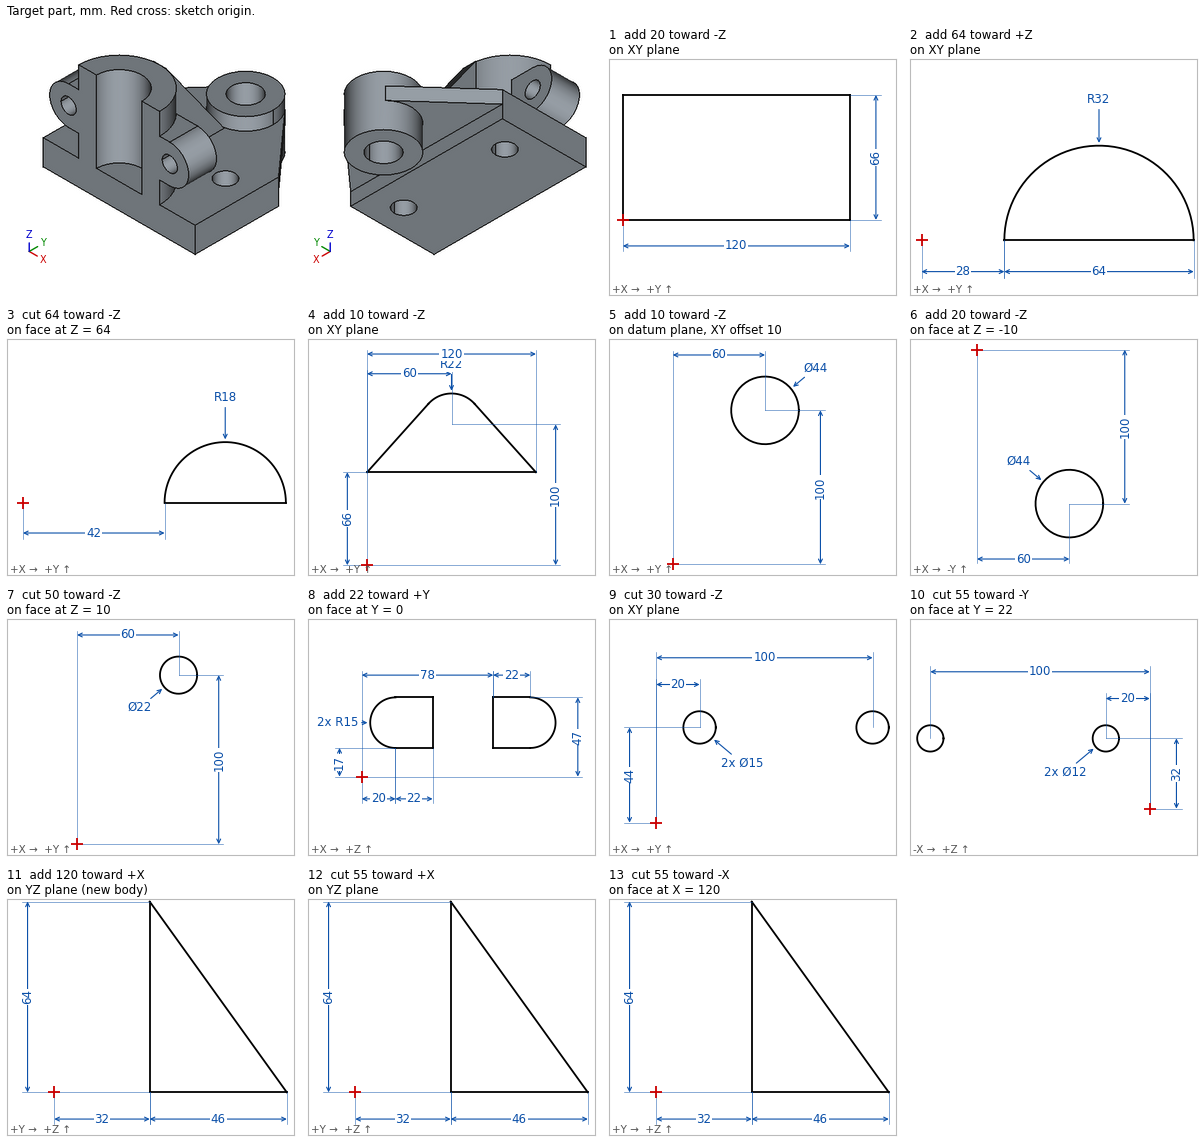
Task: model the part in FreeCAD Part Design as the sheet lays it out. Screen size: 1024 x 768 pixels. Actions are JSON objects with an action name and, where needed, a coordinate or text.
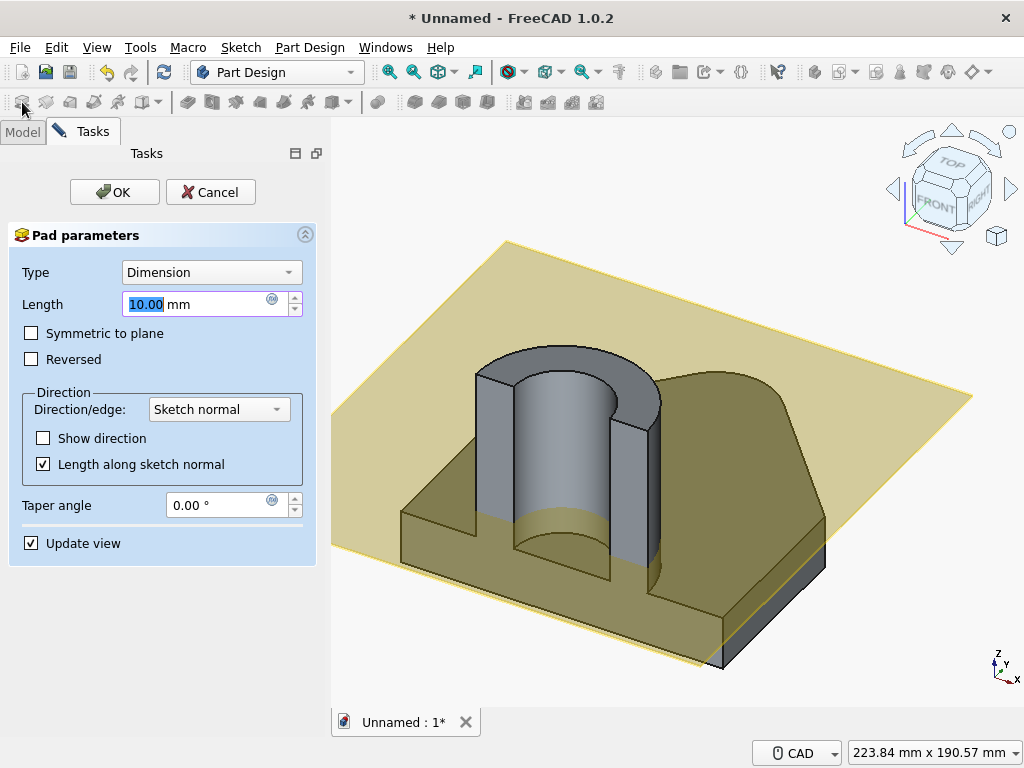
{"action": "type", "text": "10"}
{"action": "key", "text": "Tab"}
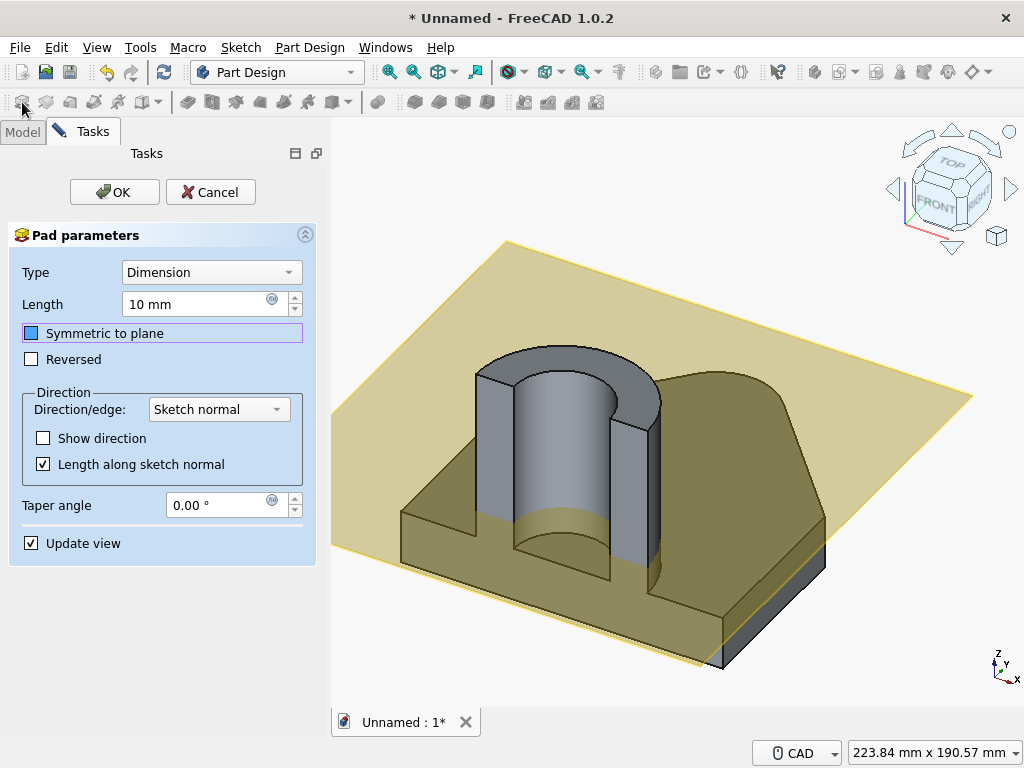
{"action": "left_click", "coordinate": [30, 359]}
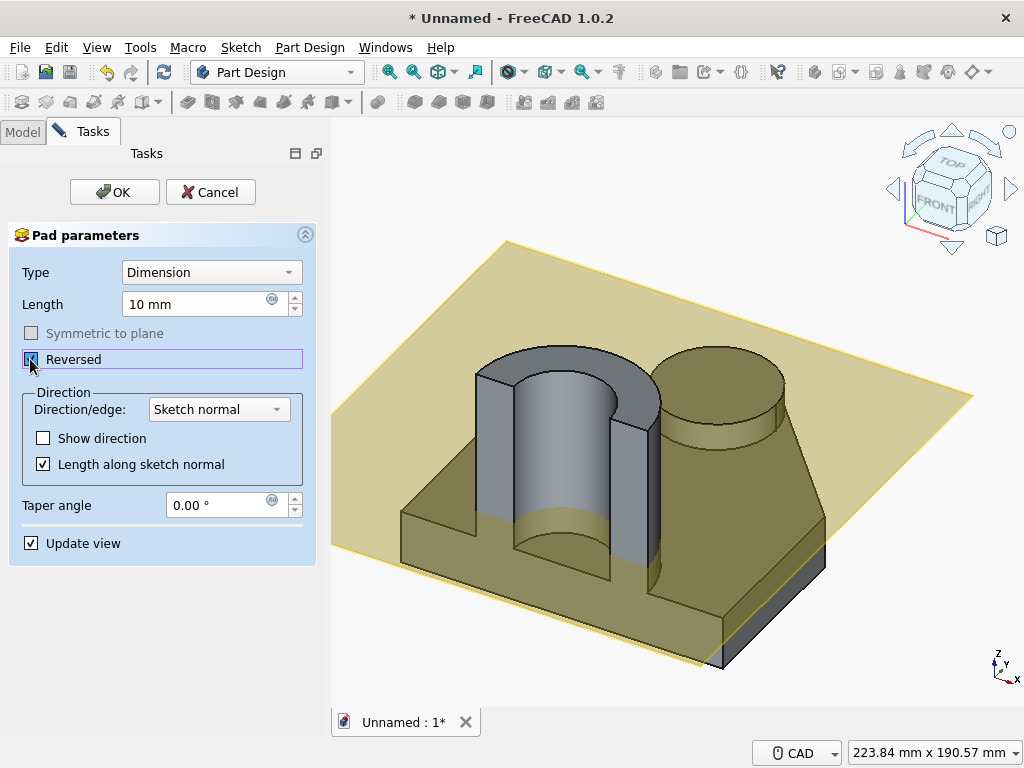
{"action": "left_click", "coordinate": [115, 192]}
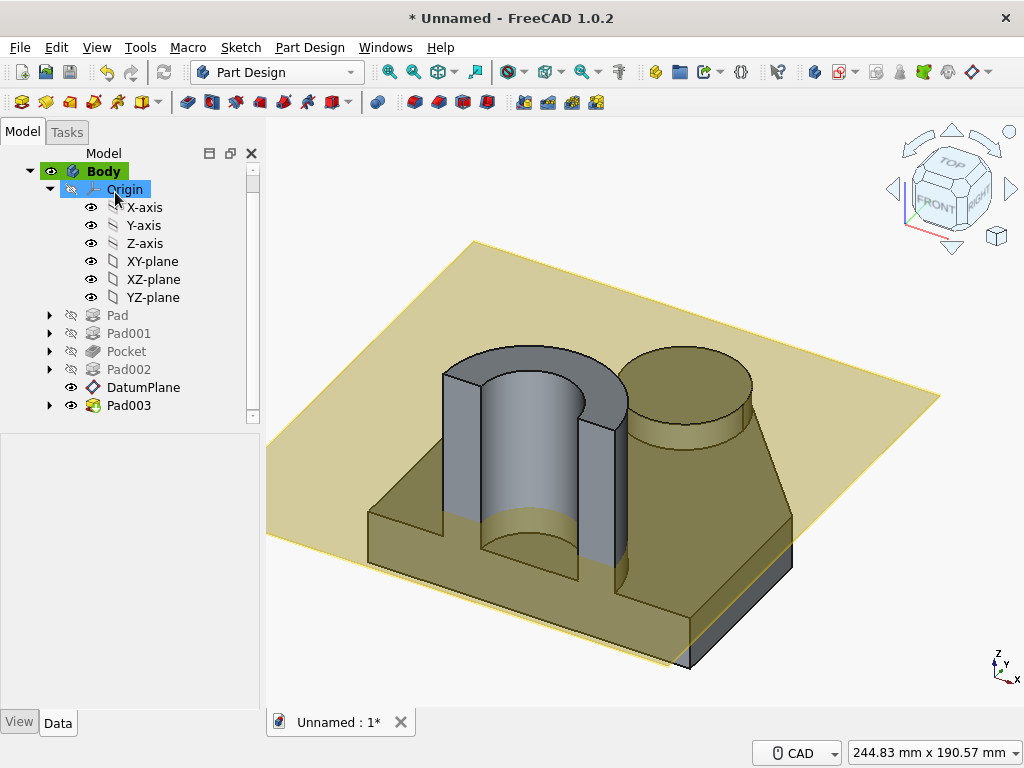
{"action": "left_click", "coordinate": [116, 387]}
{"action": "key", "text": "space"}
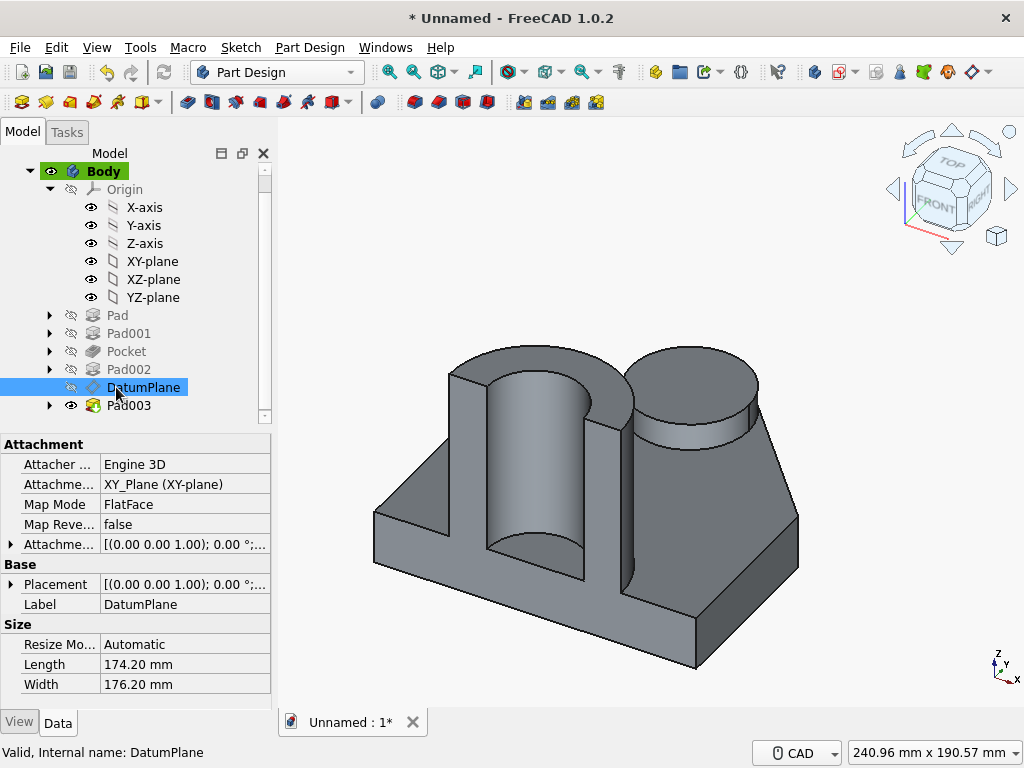
{"action": "key", "text": "5"}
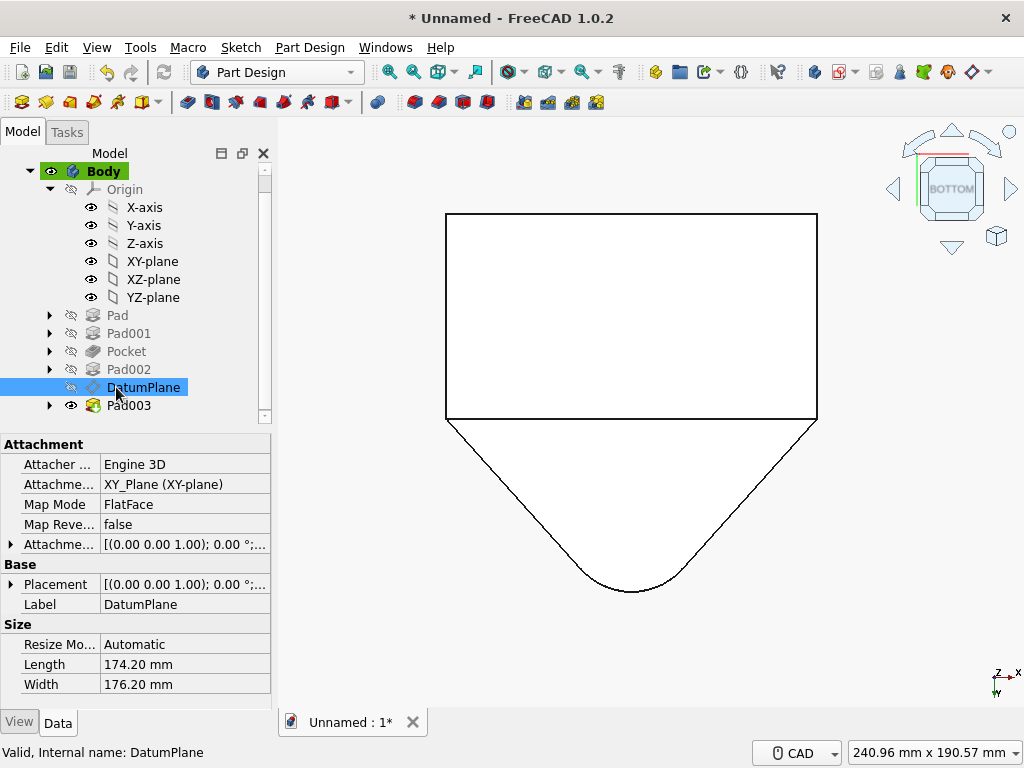
{"action": "left_click", "coordinate": [632, 504]}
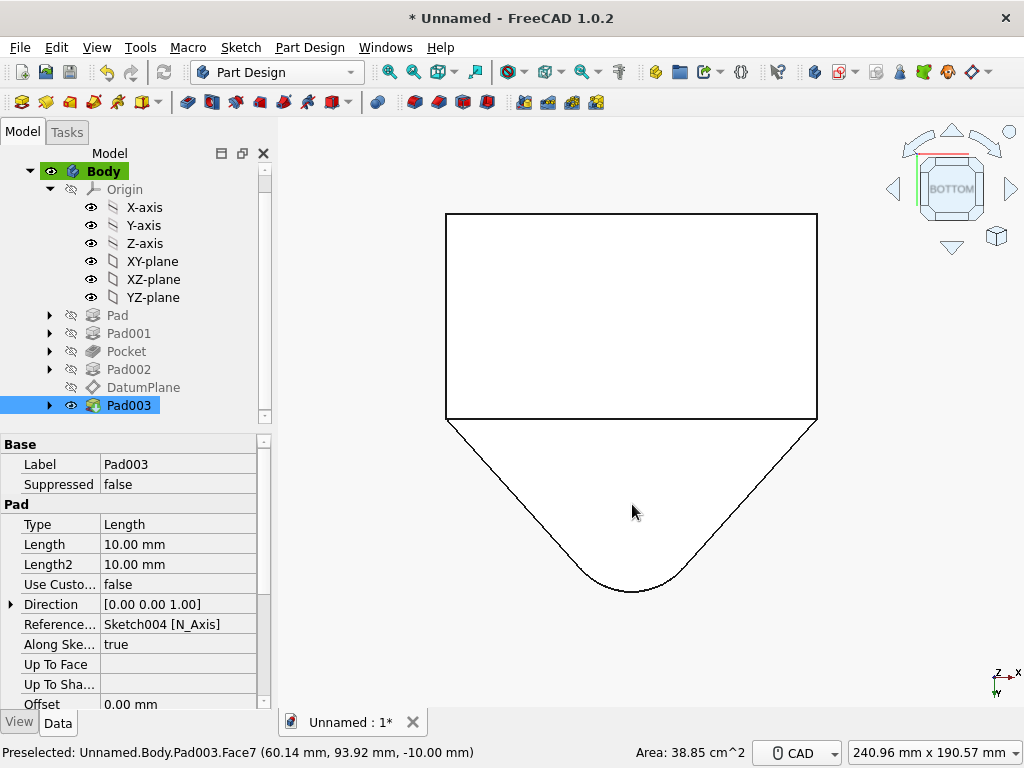
{"action": "left_click", "coordinate": [840, 72]}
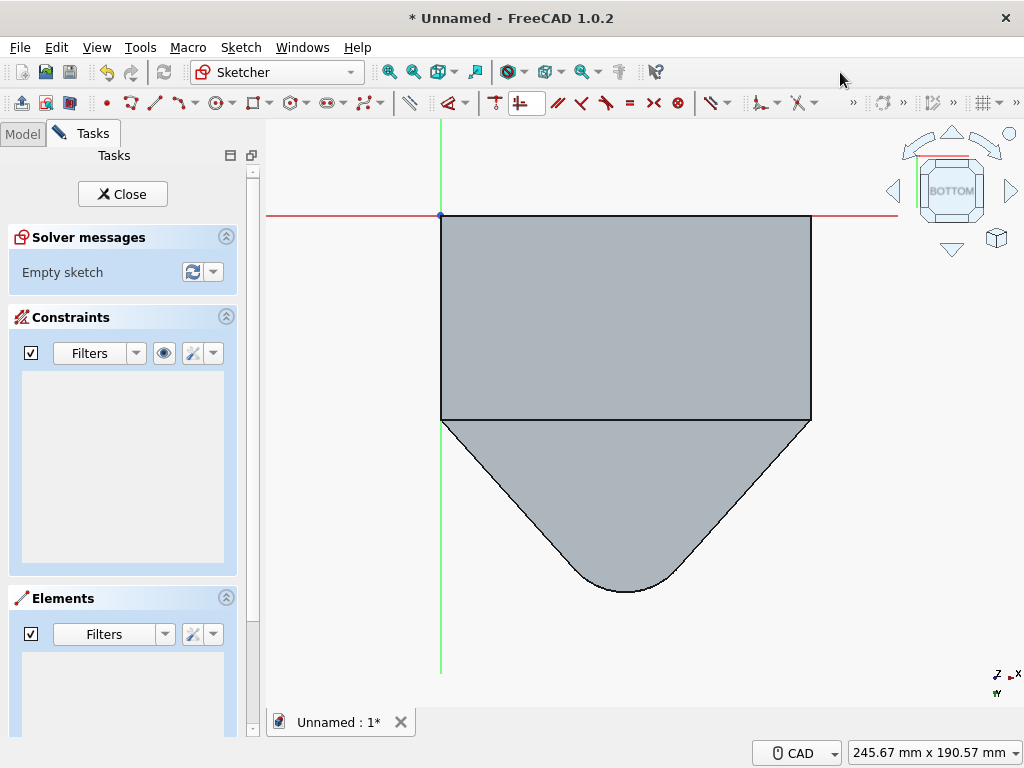
{"action": "scroll", "coordinate": [654, 589], "scroll_direction": "up", "scroll_amount": 5}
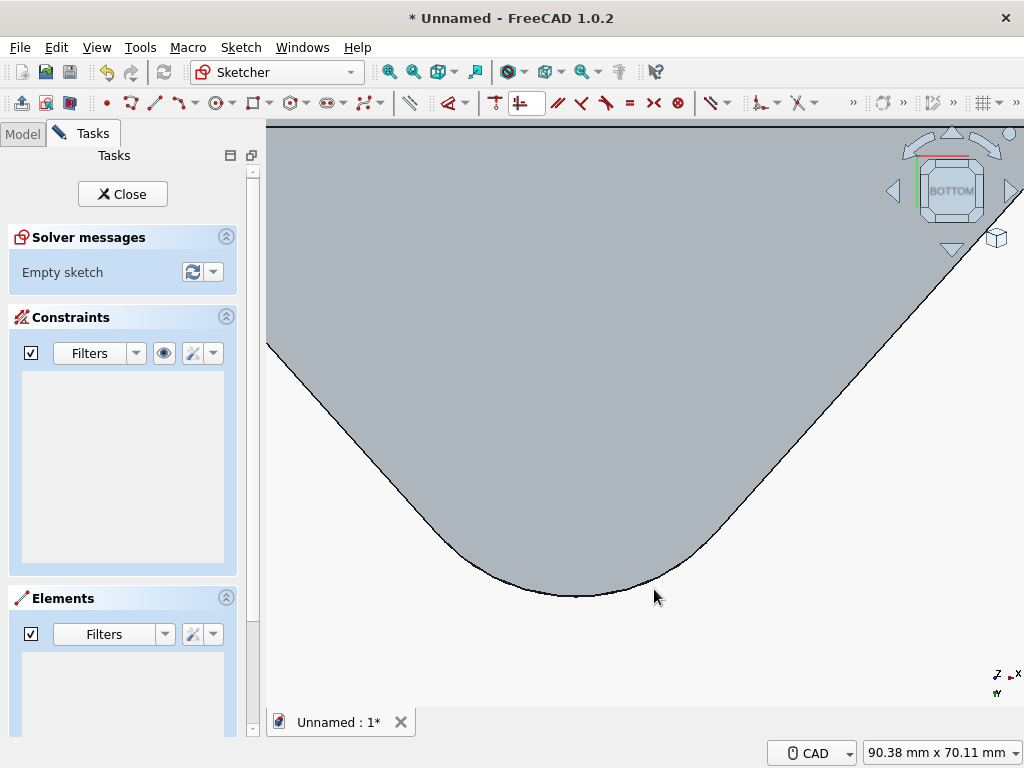
{"action": "left_click", "coordinate": [216, 104]}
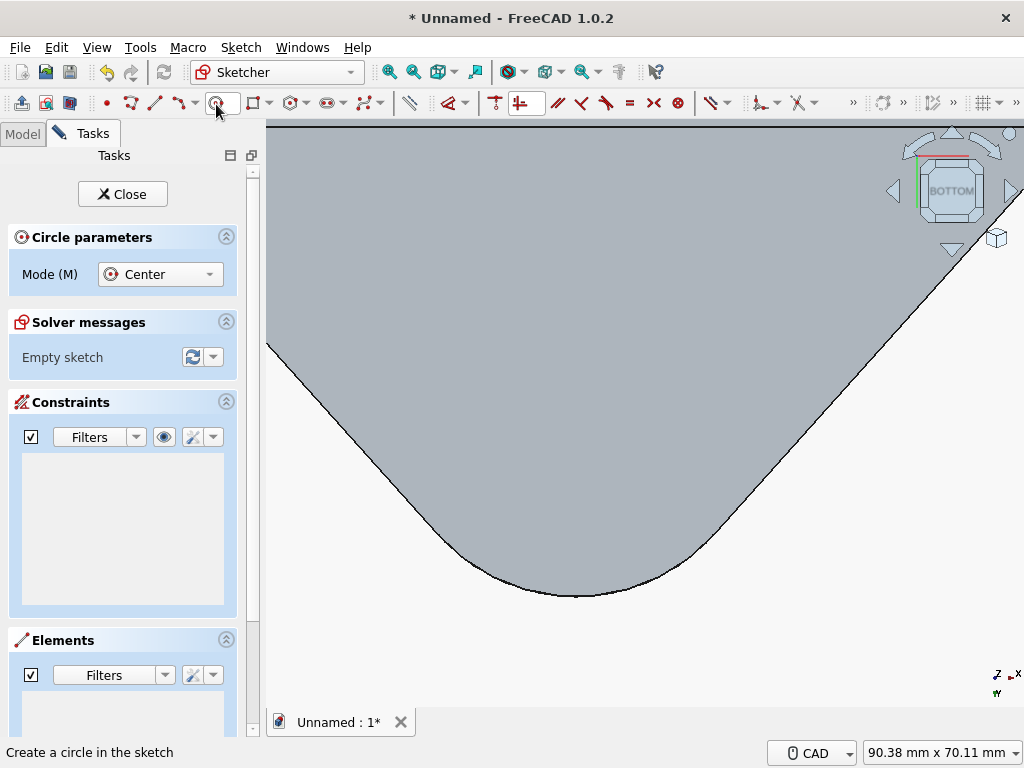
{"action": "left_click", "coordinate": [576, 412]}
{"action": "left_click", "coordinate": [707, 282]}
{"action": "key", "text": "Escape"}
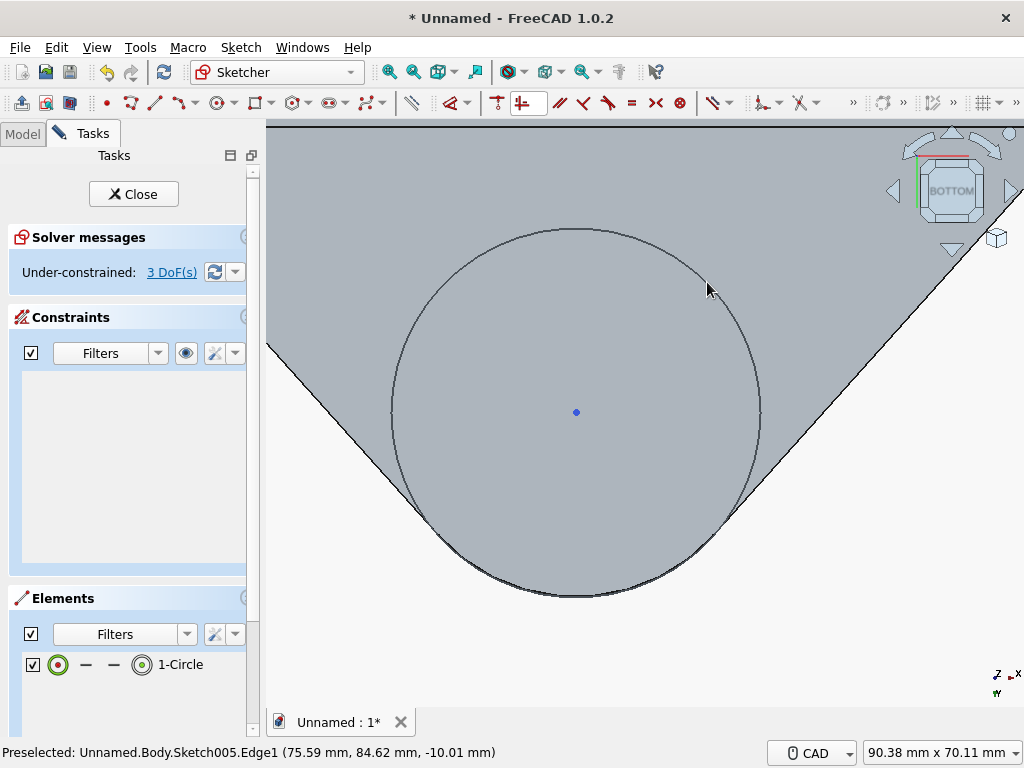
{"action": "left_click", "coordinate": [450, 104]}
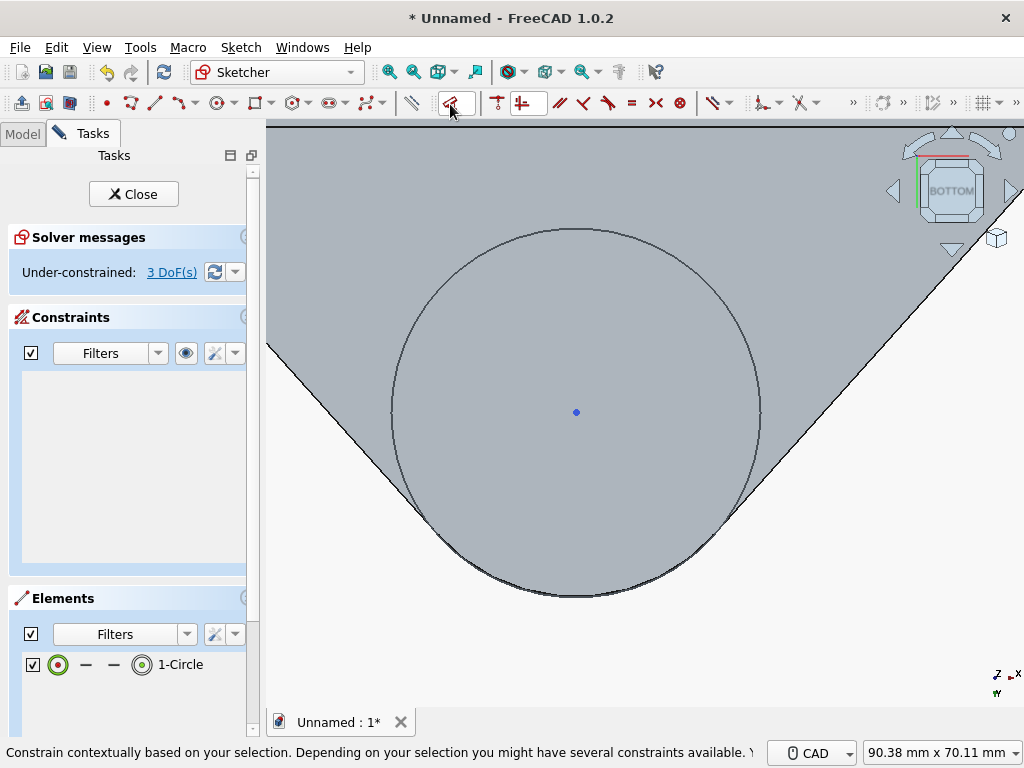
{"action": "left_click", "coordinate": [706, 282]}
{"action": "left_click", "coordinate": [729, 259]}